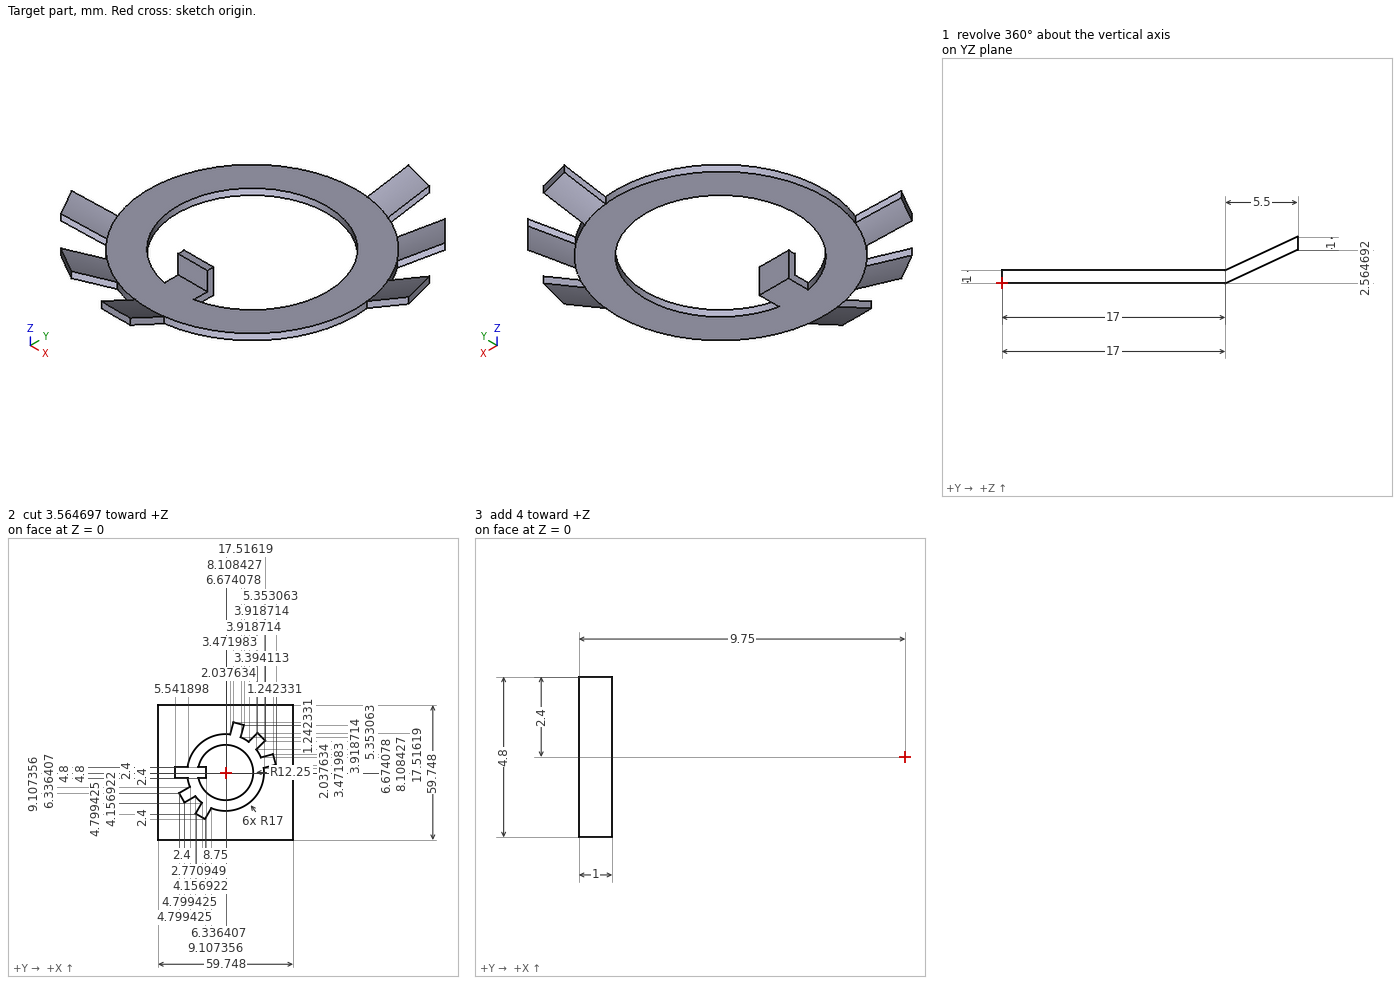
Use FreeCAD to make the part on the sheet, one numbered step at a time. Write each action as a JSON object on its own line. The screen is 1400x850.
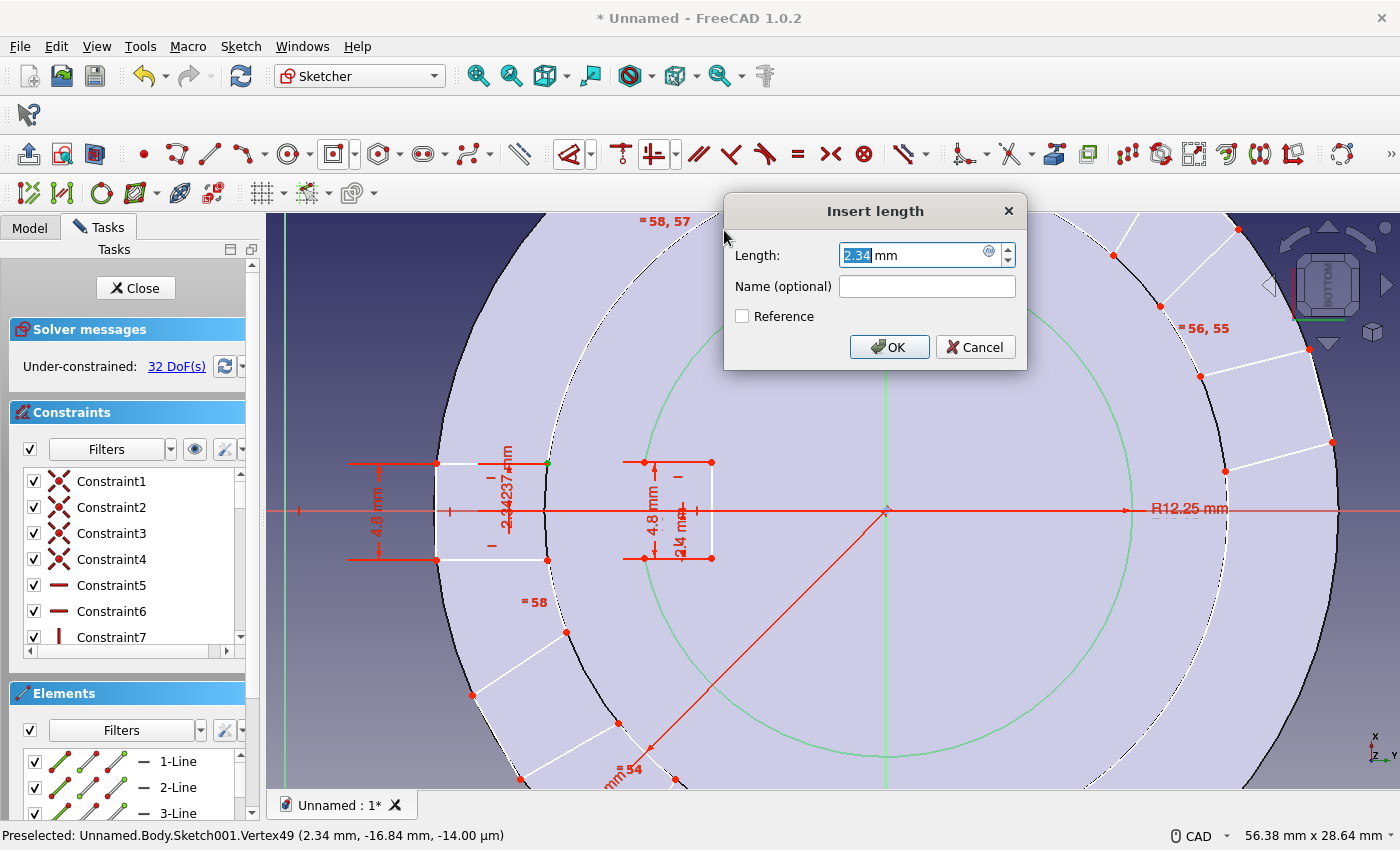
{"action": "type", "text": "2.4"}
{"action": "key", "text": "Return"}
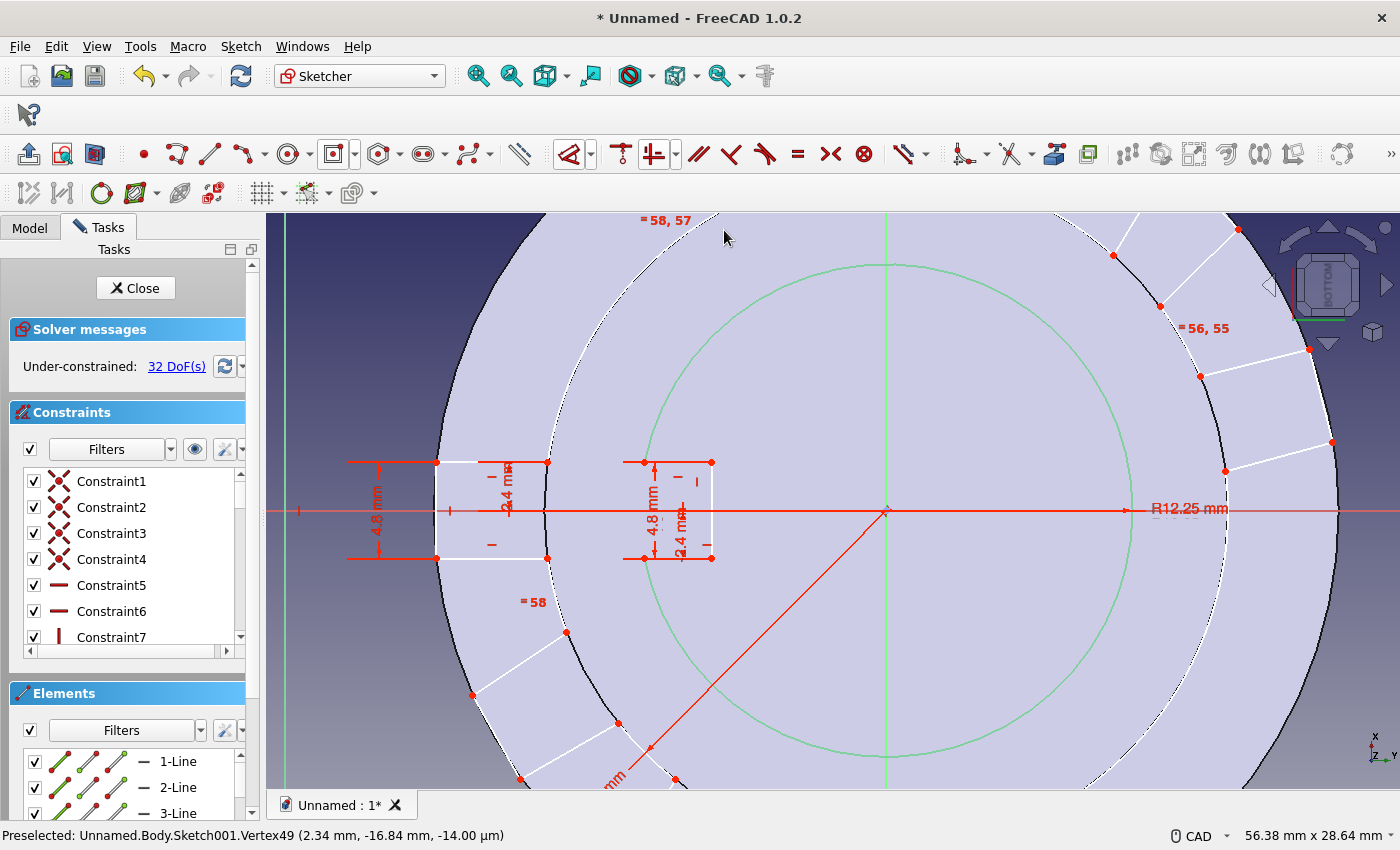
{"action": "left_click", "coordinate": [487, 721]}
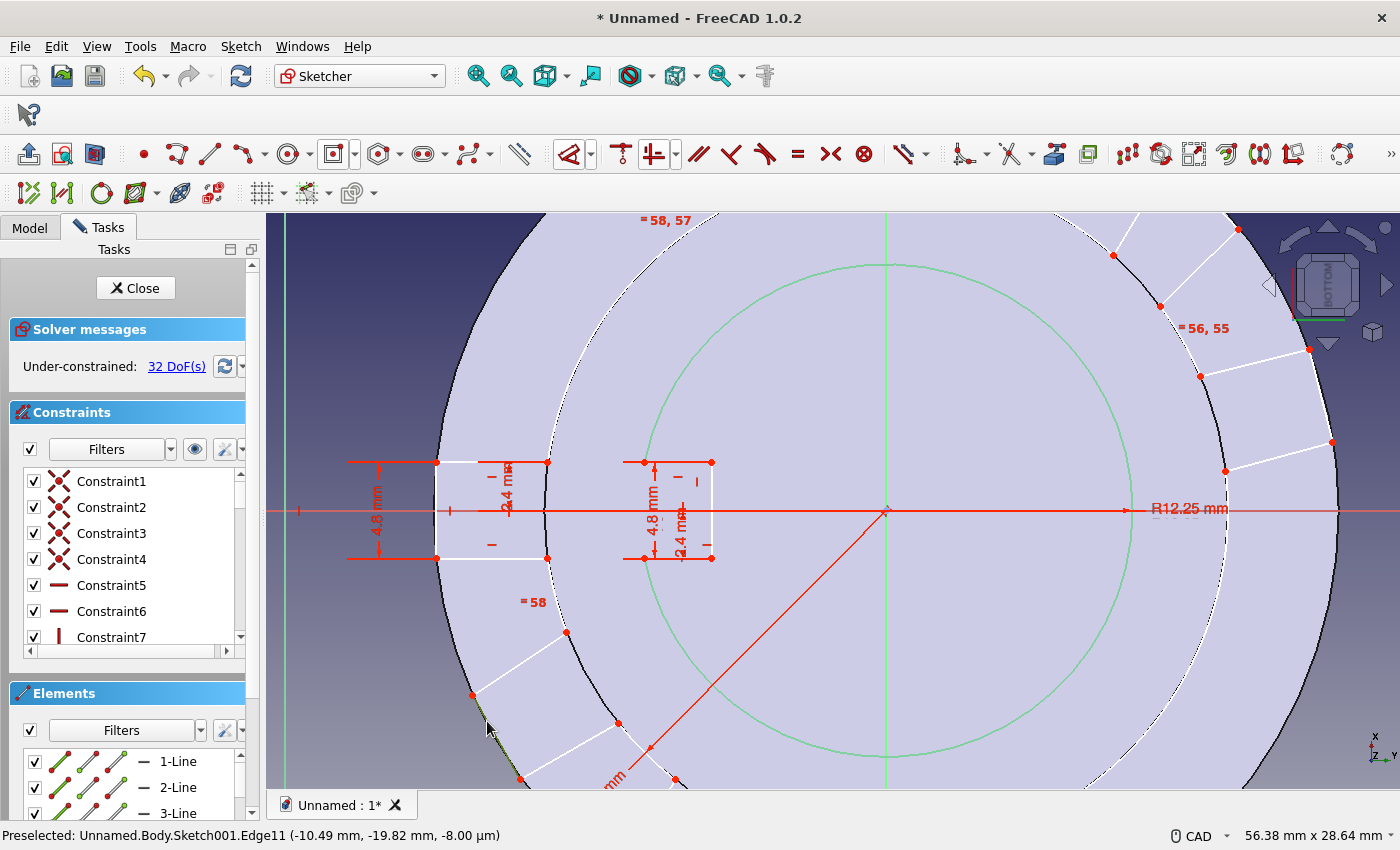
{"action": "key", "text": "l"}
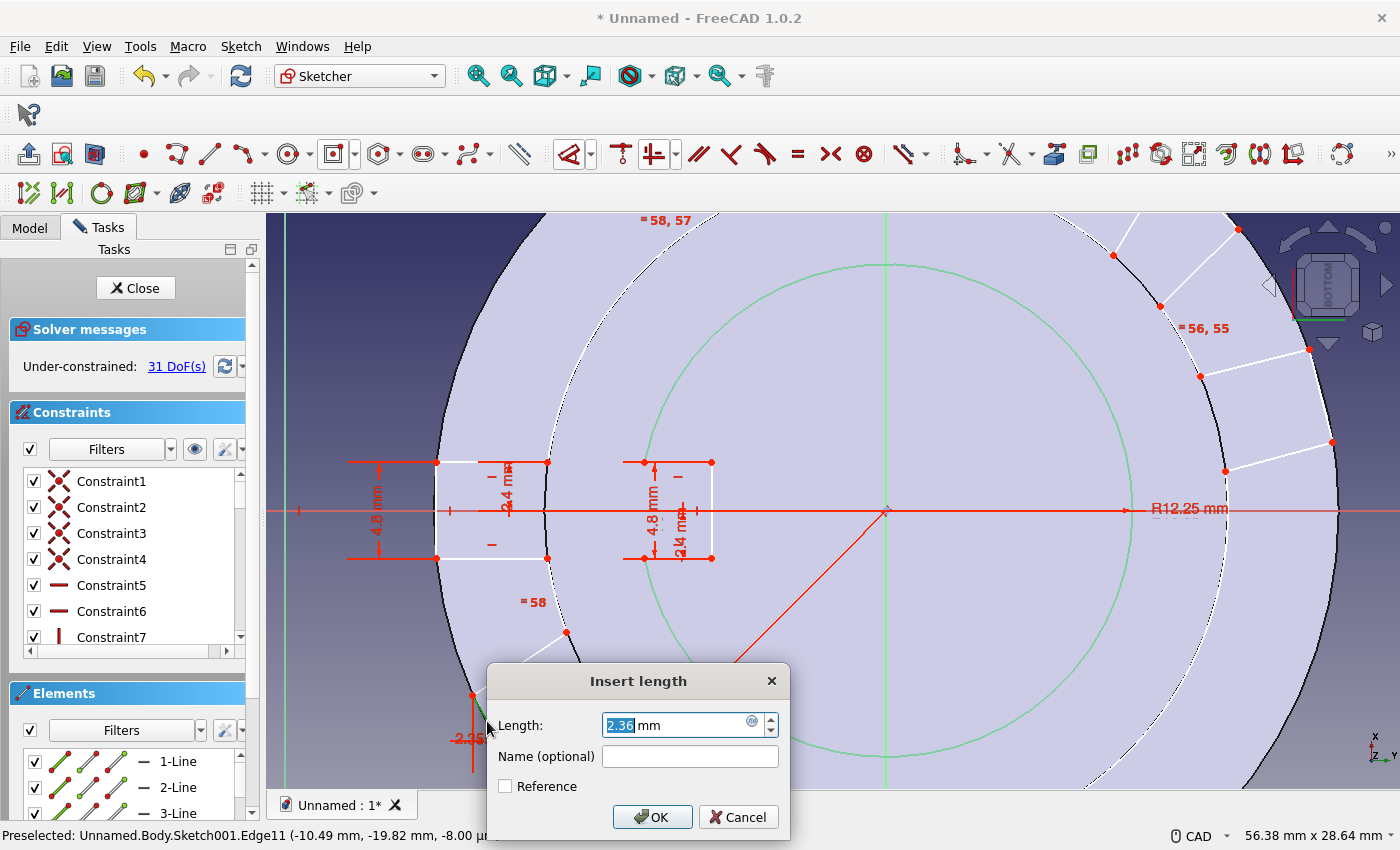
{"action": "type", "text": "2.4"}
{"action": "key", "text": "Return"}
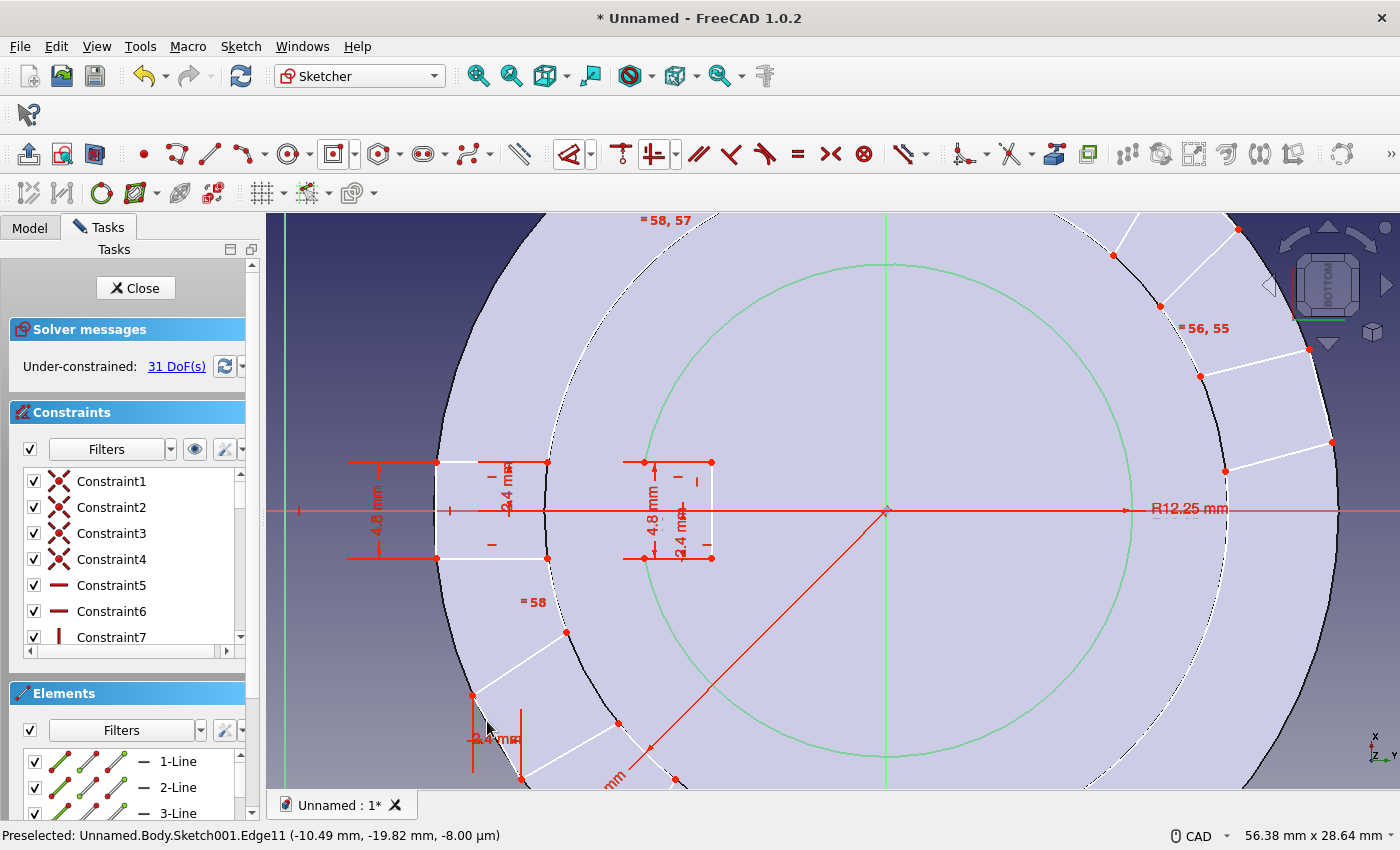
{"action": "scroll", "coordinate": [712, 497], "scroll_direction": "down", "scroll_amount": 6}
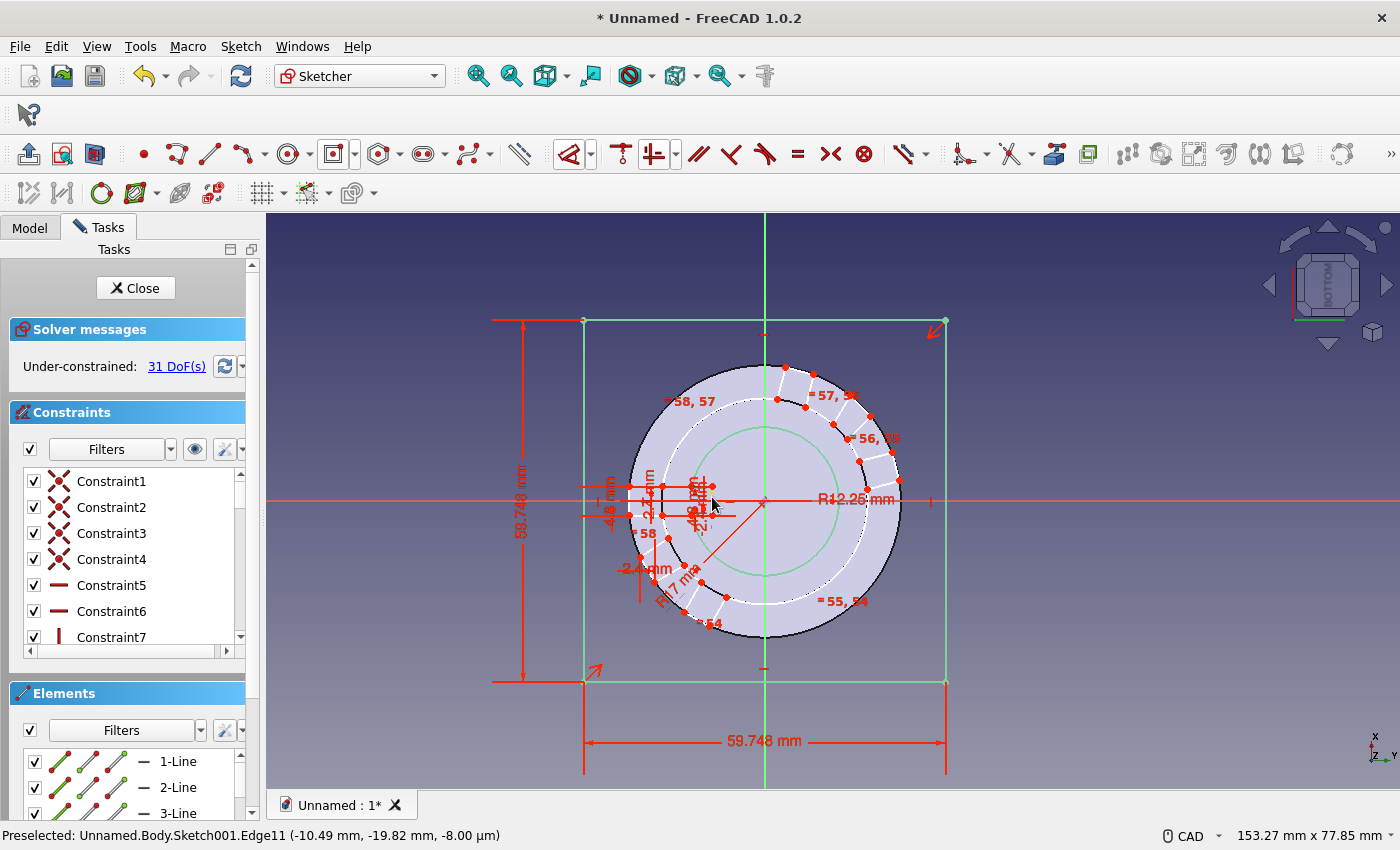
{"action": "scroll", "coordinate": [692, 617], "scroll_direction": "up", "scroll_amount": 6}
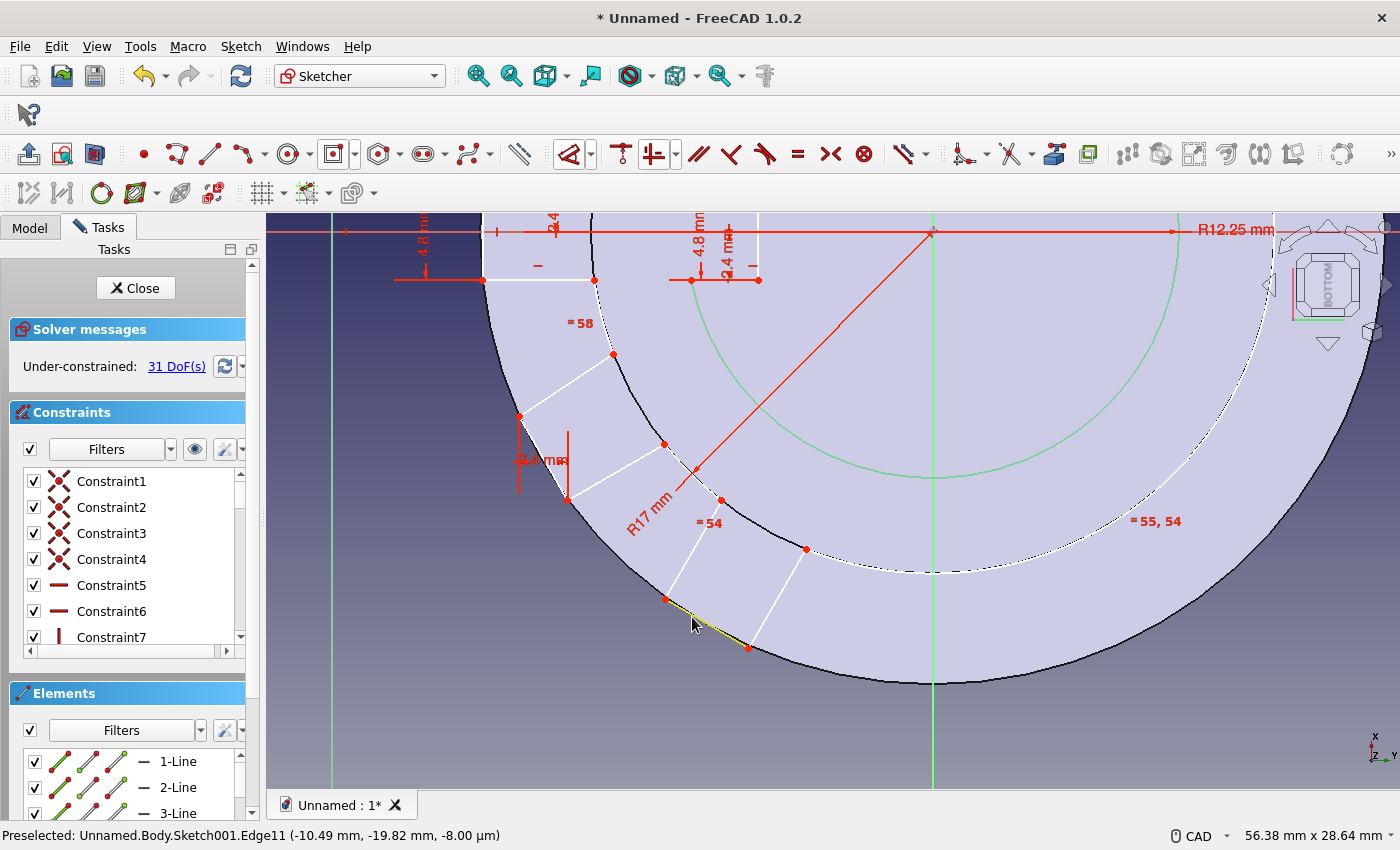
{"action": "left_click", "coordinate": [690, 614]}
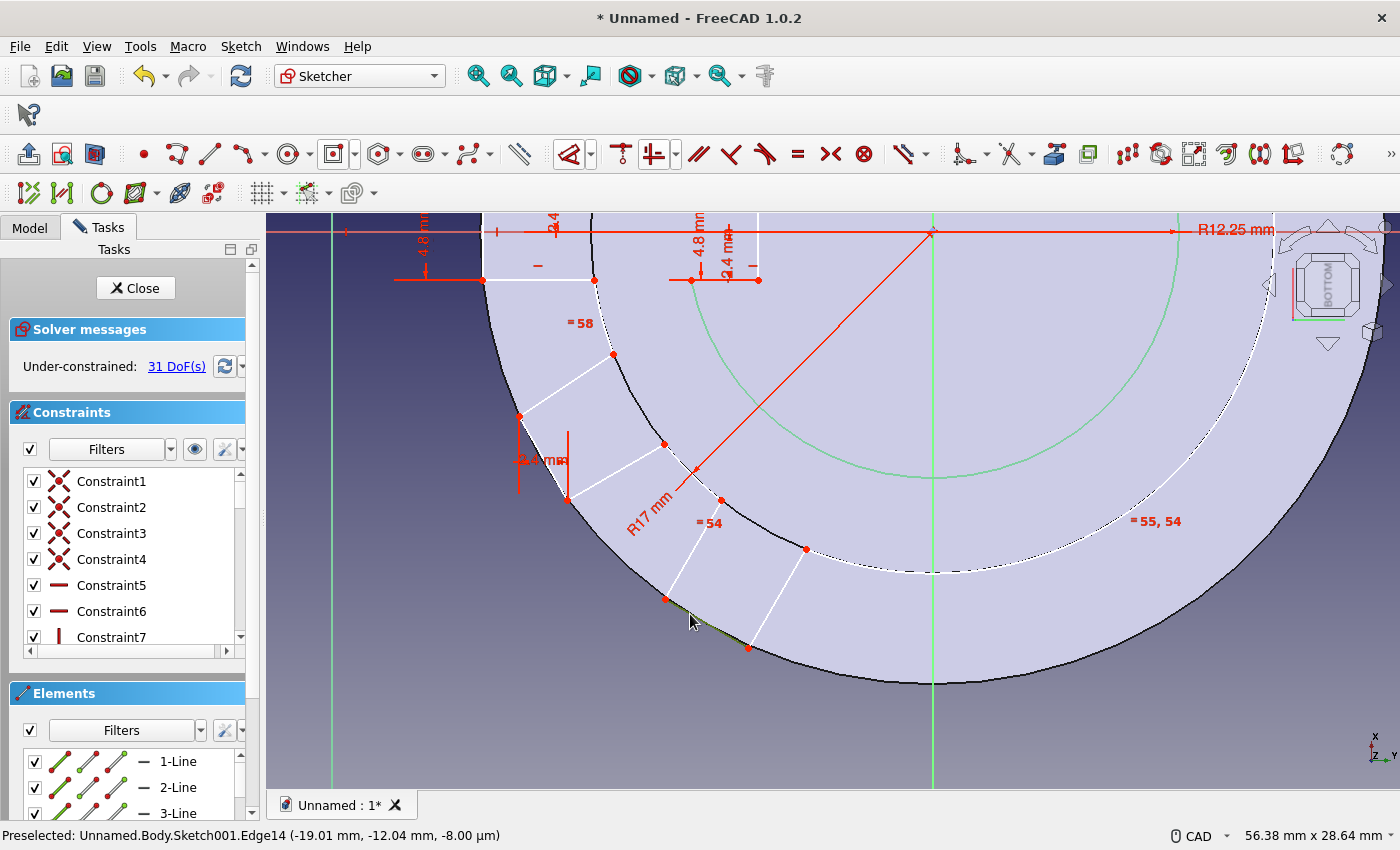
{"action": "key", "text": "i"}